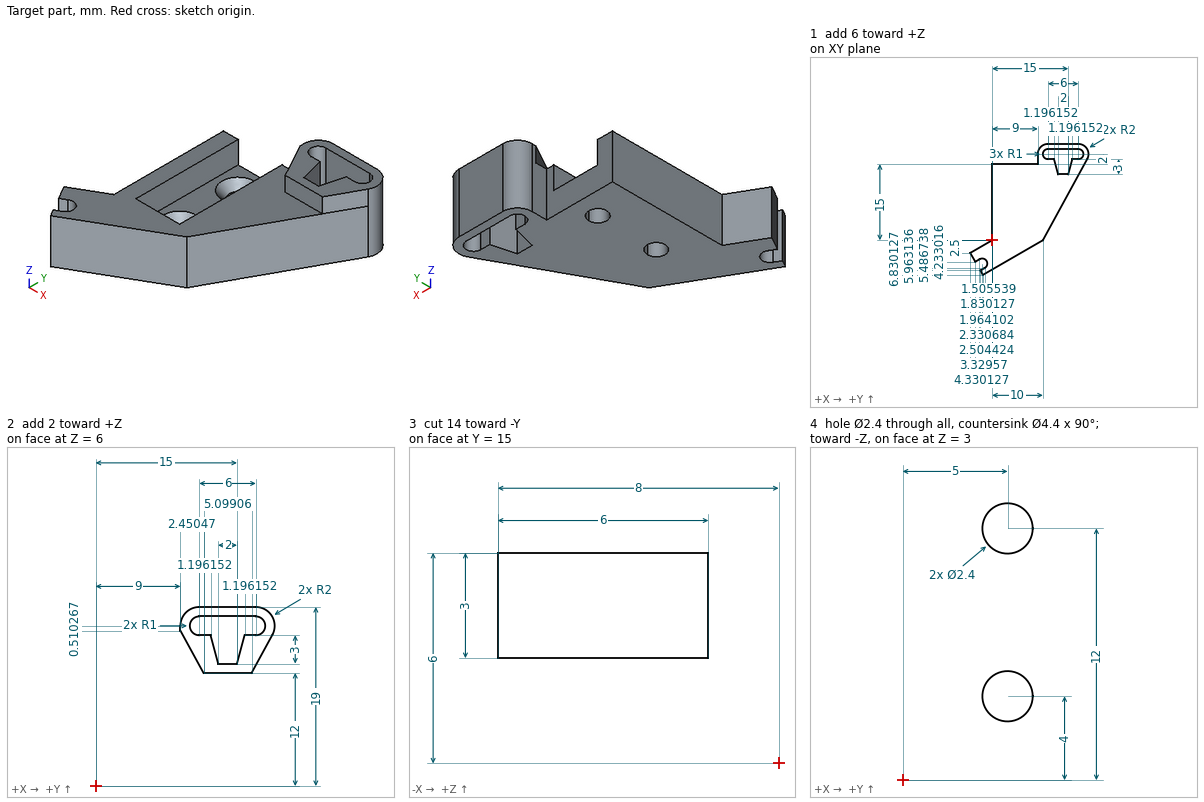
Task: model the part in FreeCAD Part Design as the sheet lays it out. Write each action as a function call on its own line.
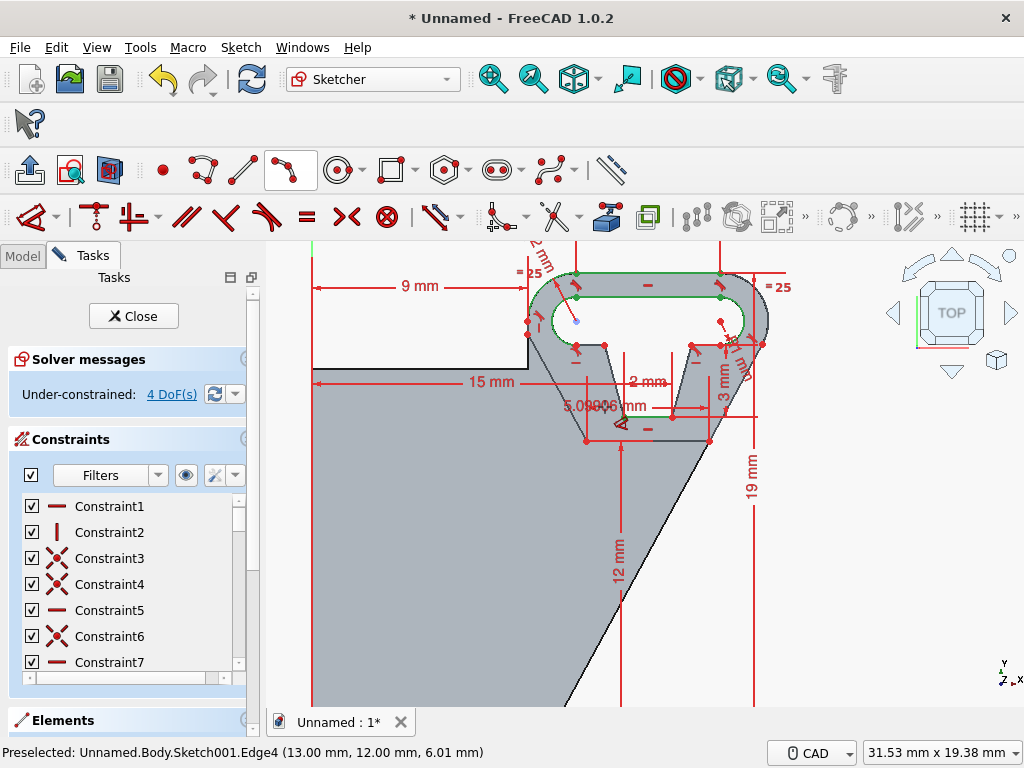
scroll(528, 328, up, 6)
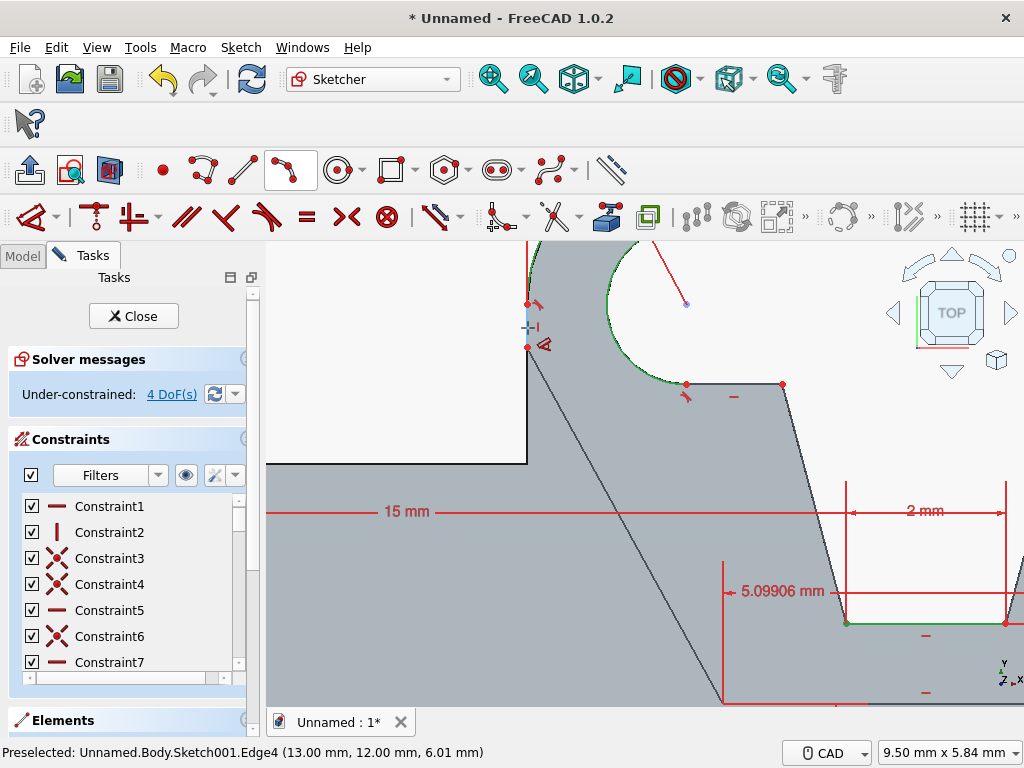
click(527, 326)
click(493, 326)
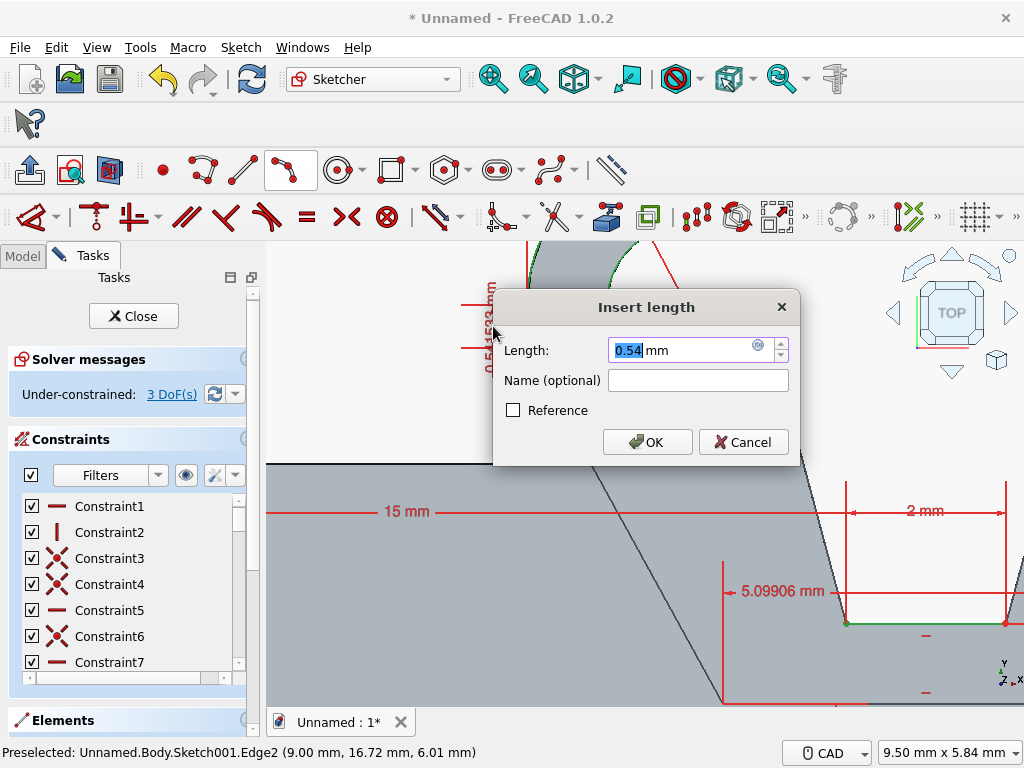
text(0.510267)
key(Return)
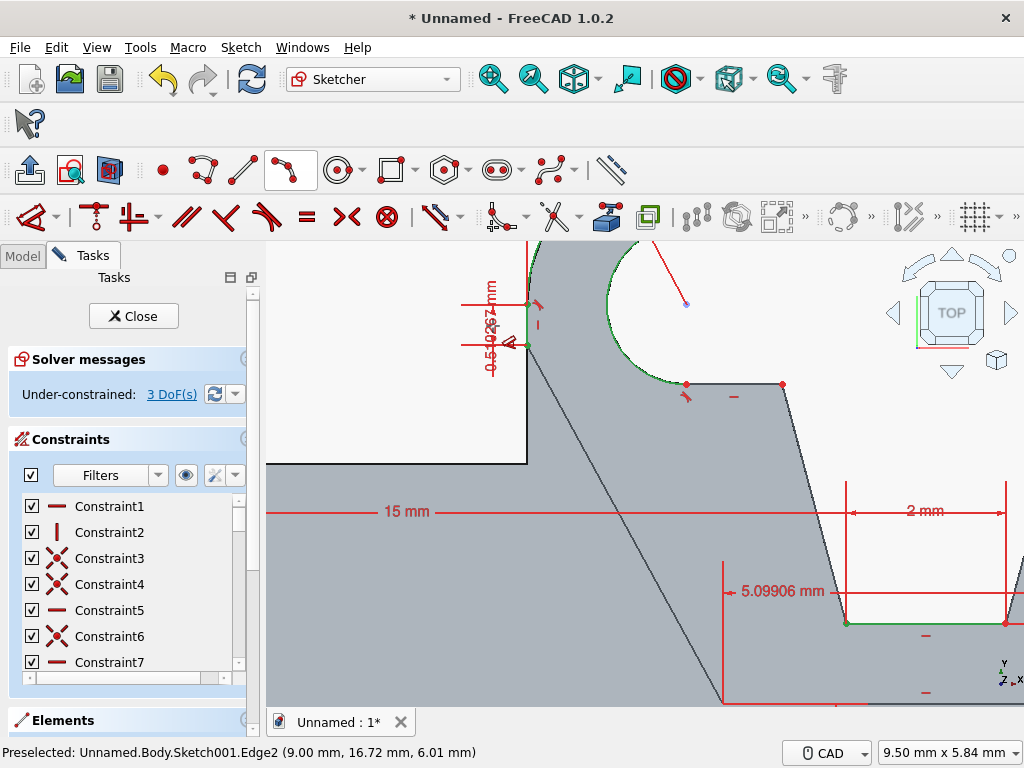
scroll(581, 365, down, 8)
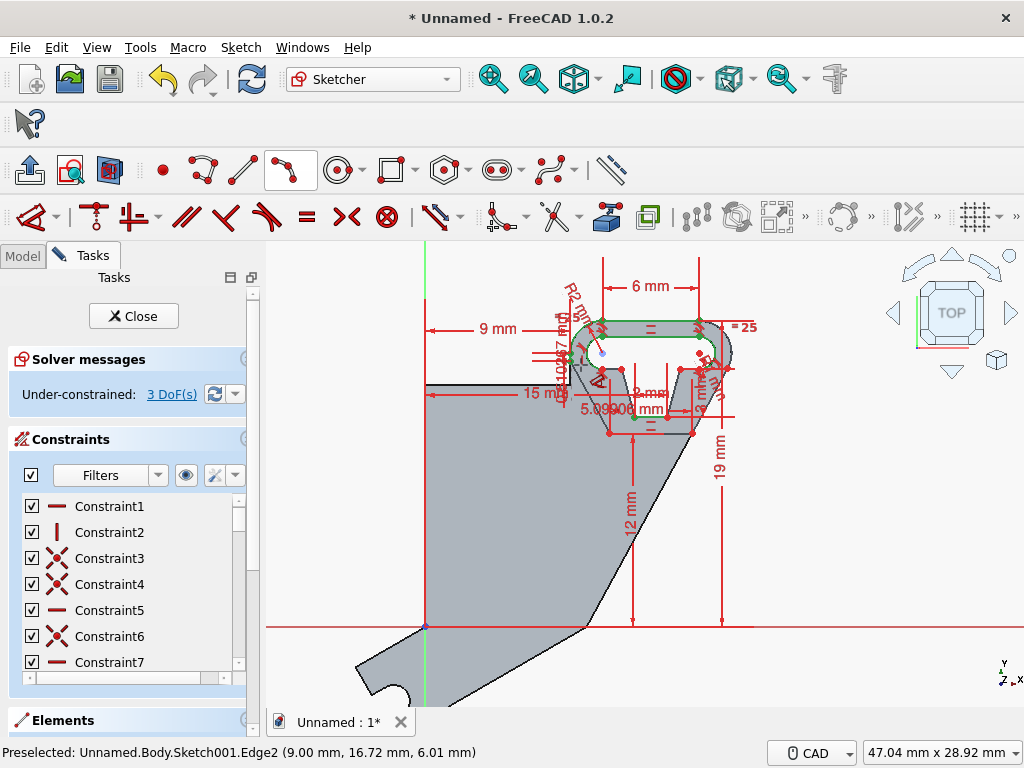
scroll(694, 369, up, 5)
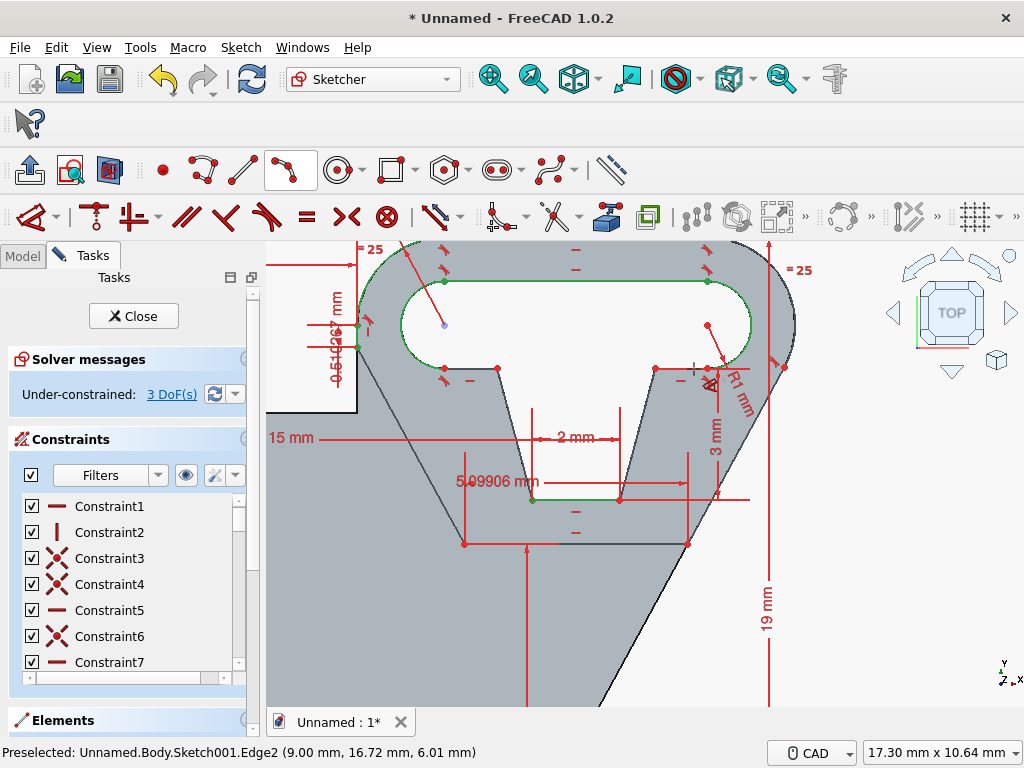
click(692, 369)
click(681, 335)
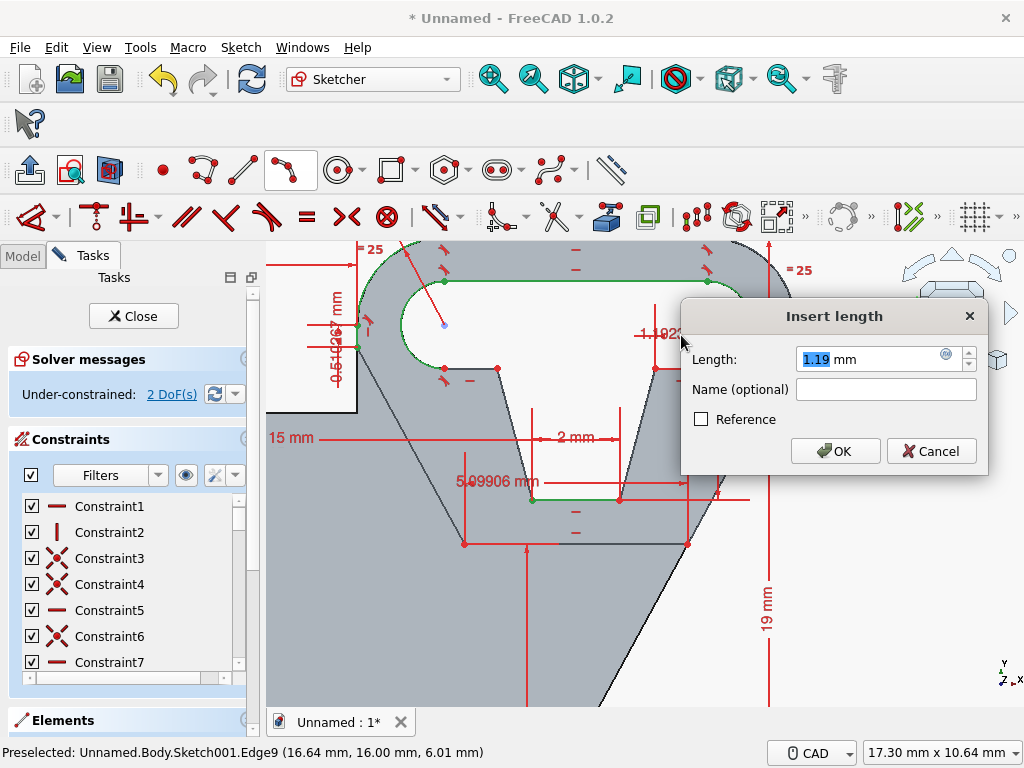
text(1.196152)
key(Return)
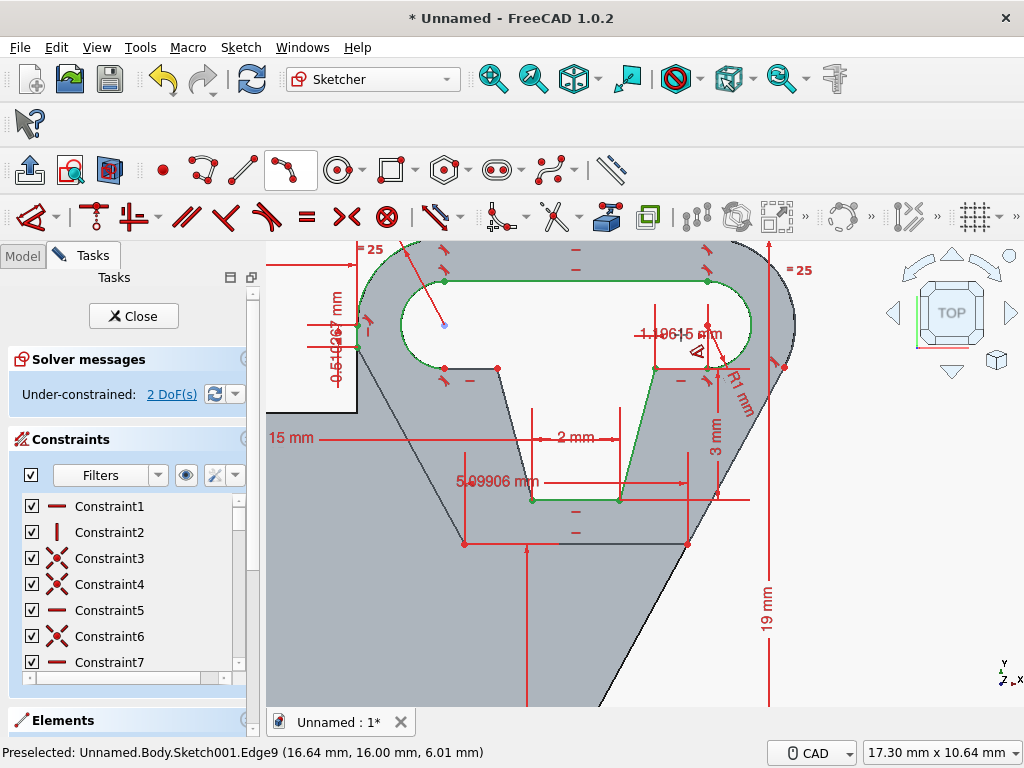
click(481, 369)
click(471, 335)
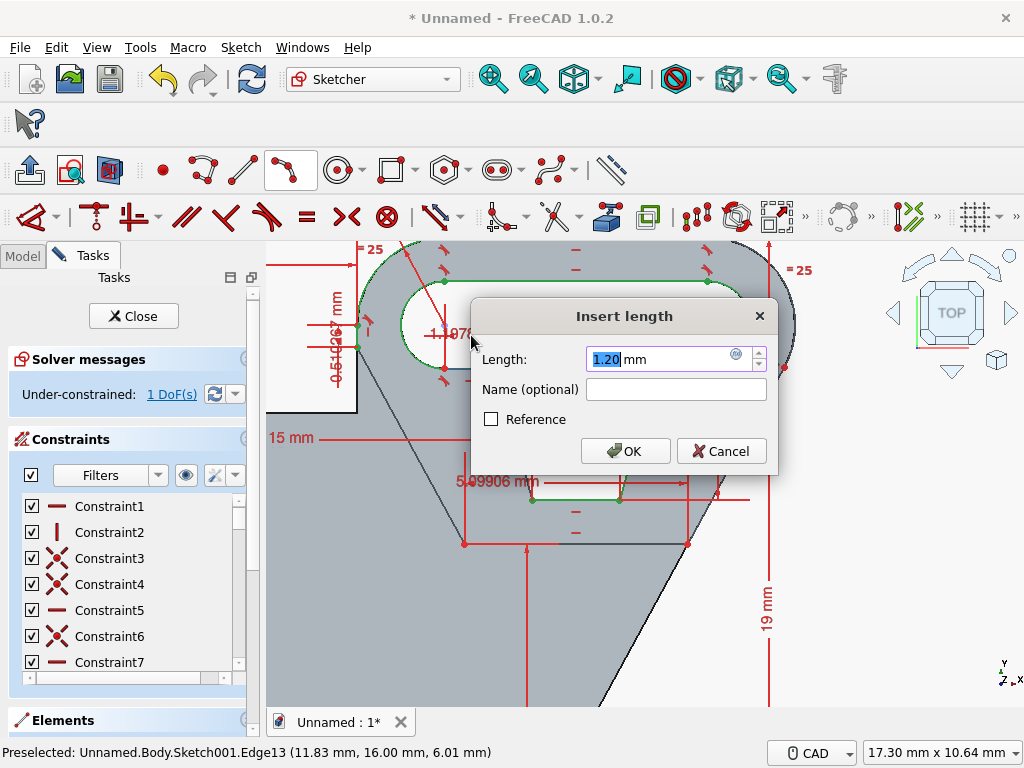
text(1.196152)
key(Return)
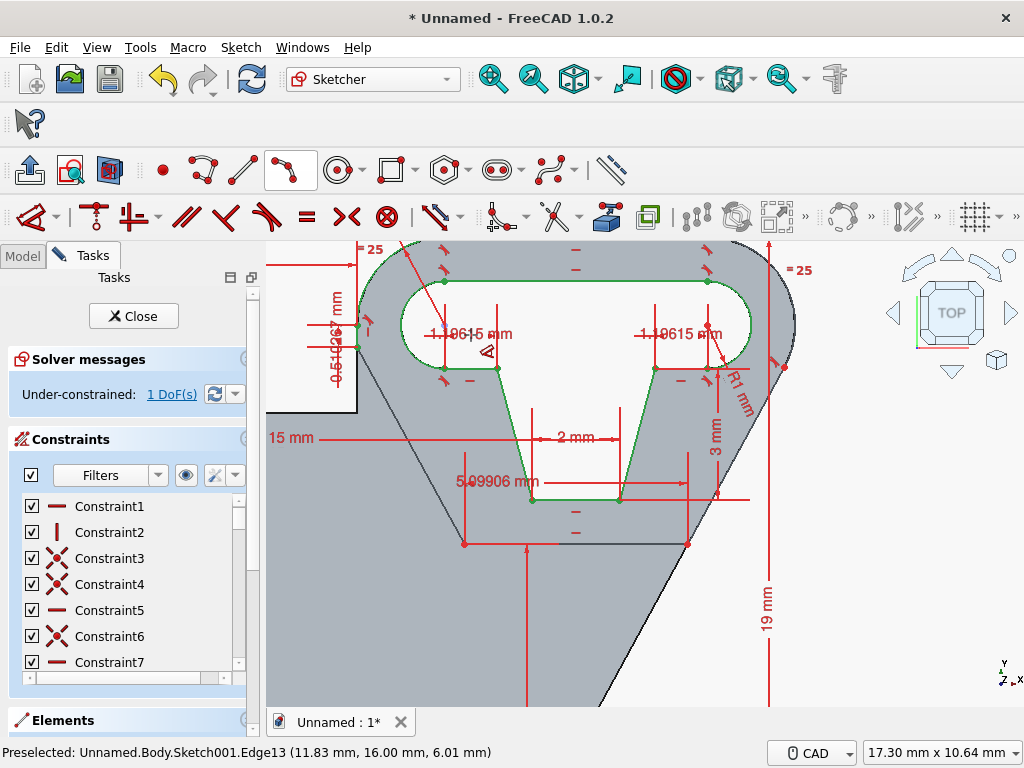
click(389, 406)
click(386, 313)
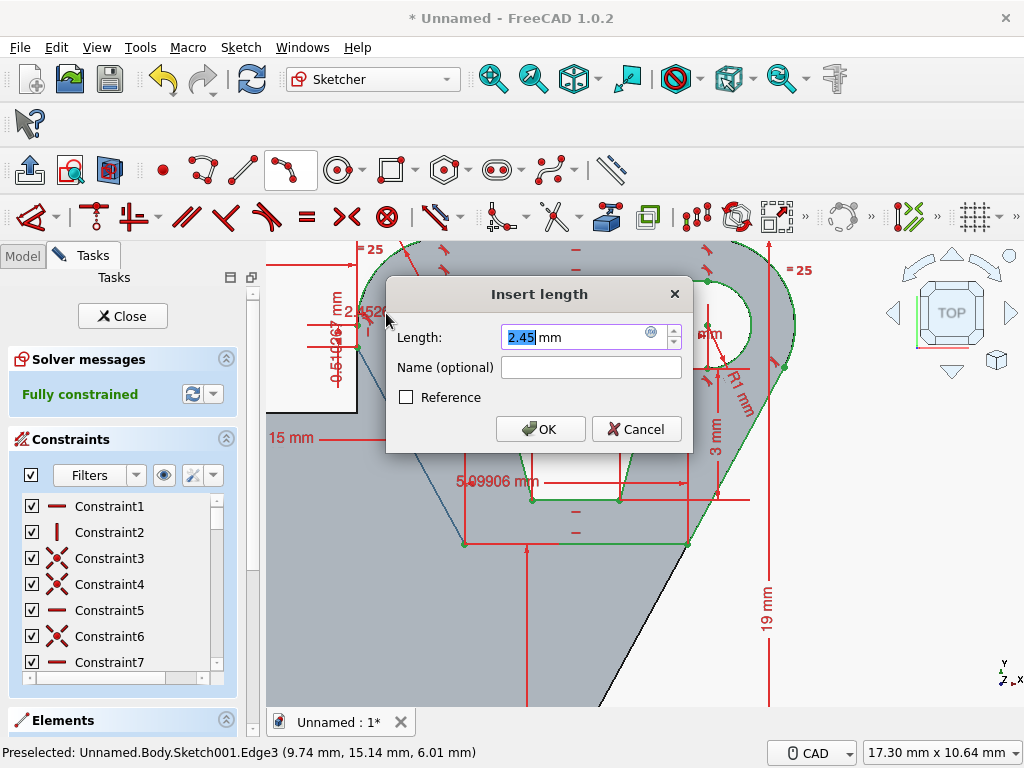
text(2.45047)
key(Return)
key(Escape)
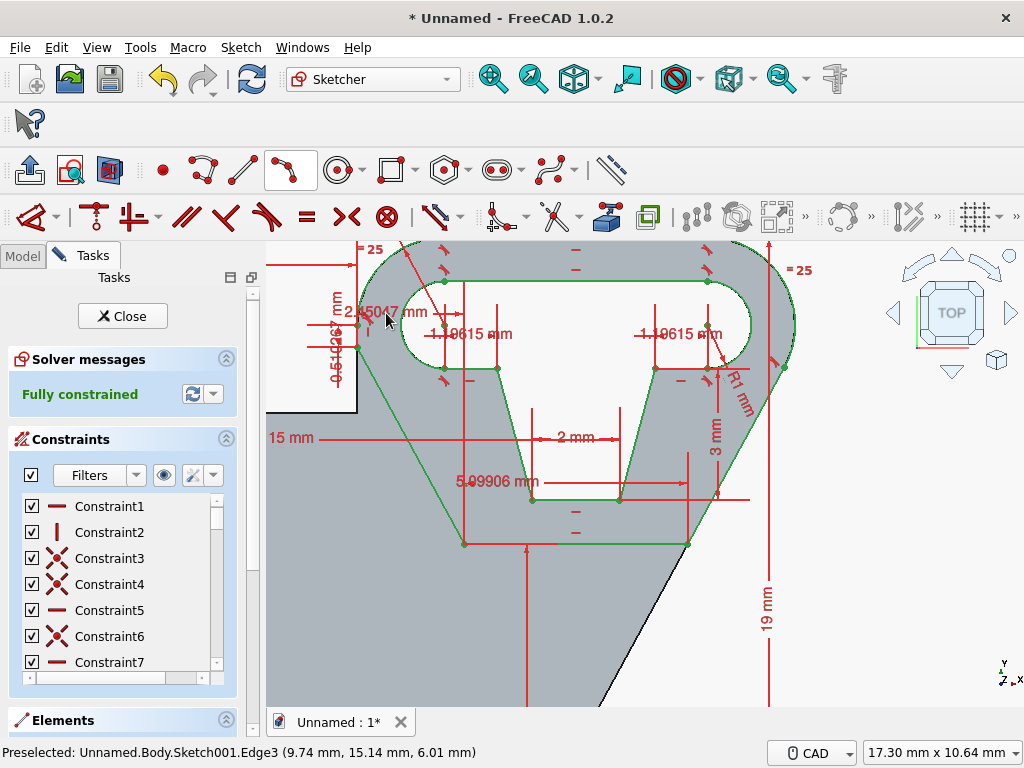
click(123, 316)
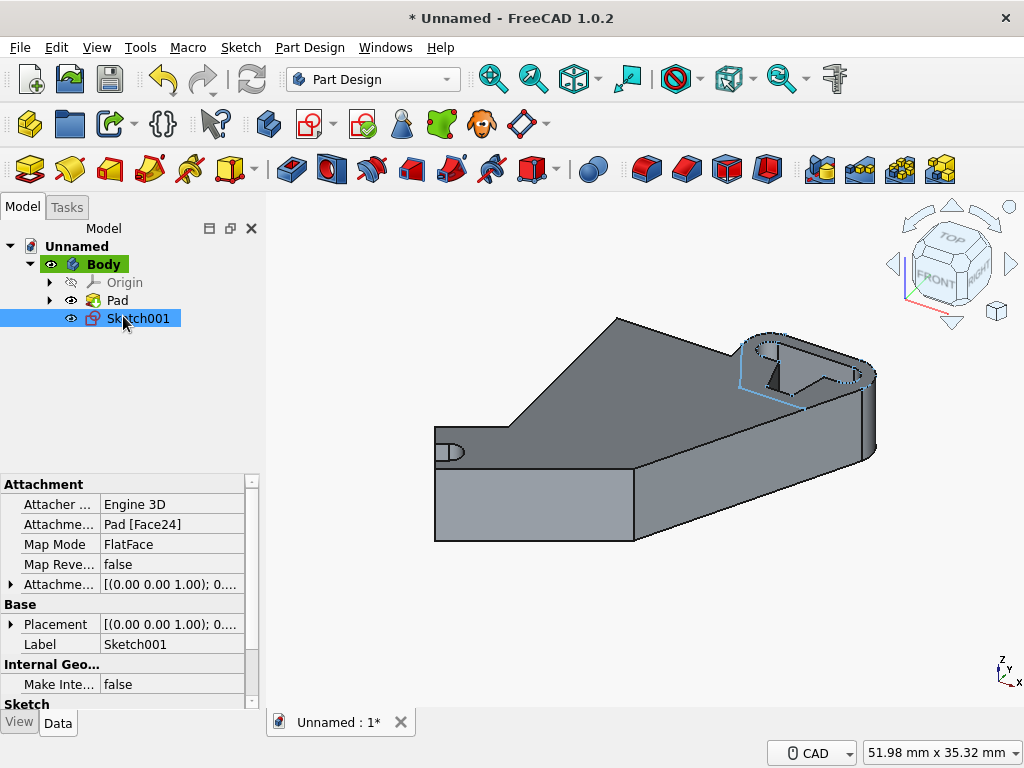
click(30, 170)